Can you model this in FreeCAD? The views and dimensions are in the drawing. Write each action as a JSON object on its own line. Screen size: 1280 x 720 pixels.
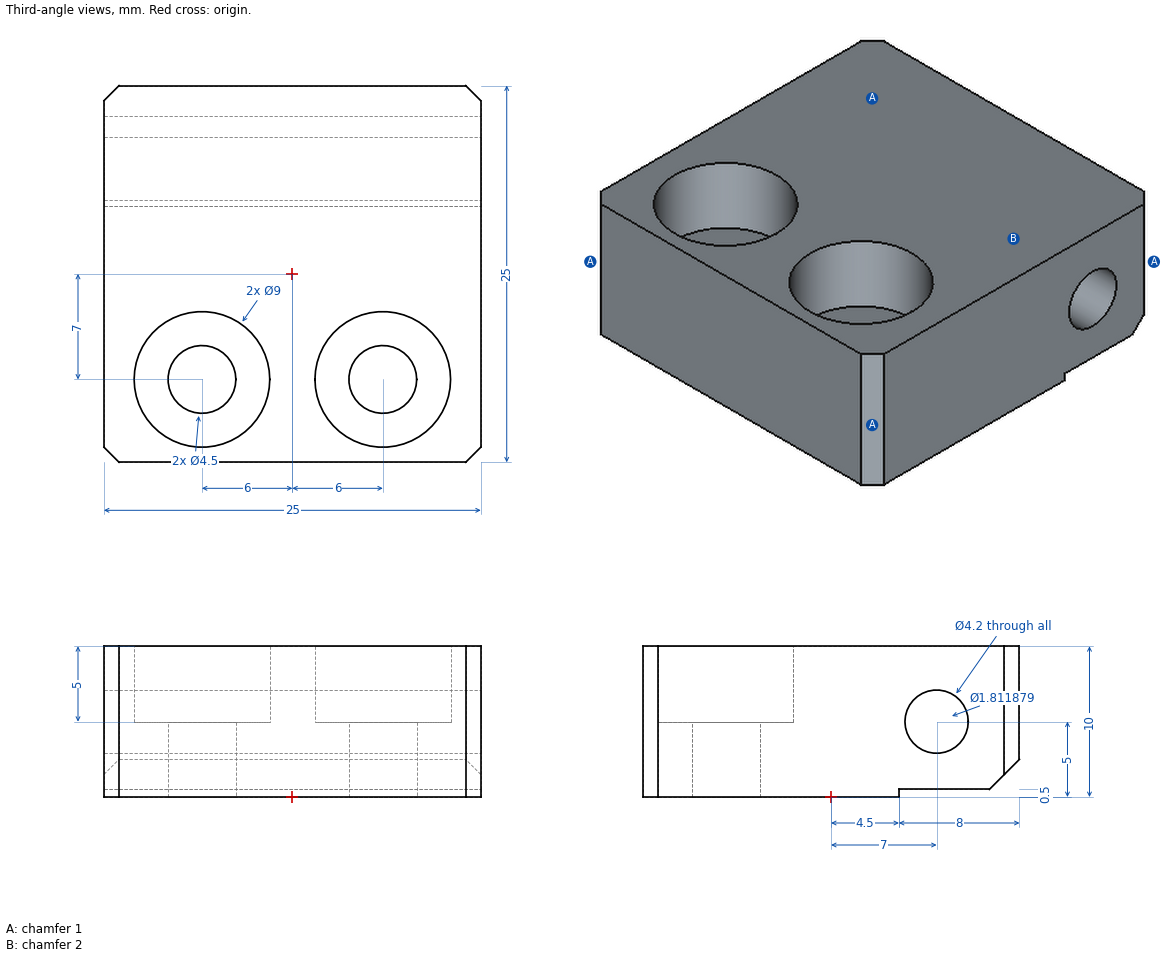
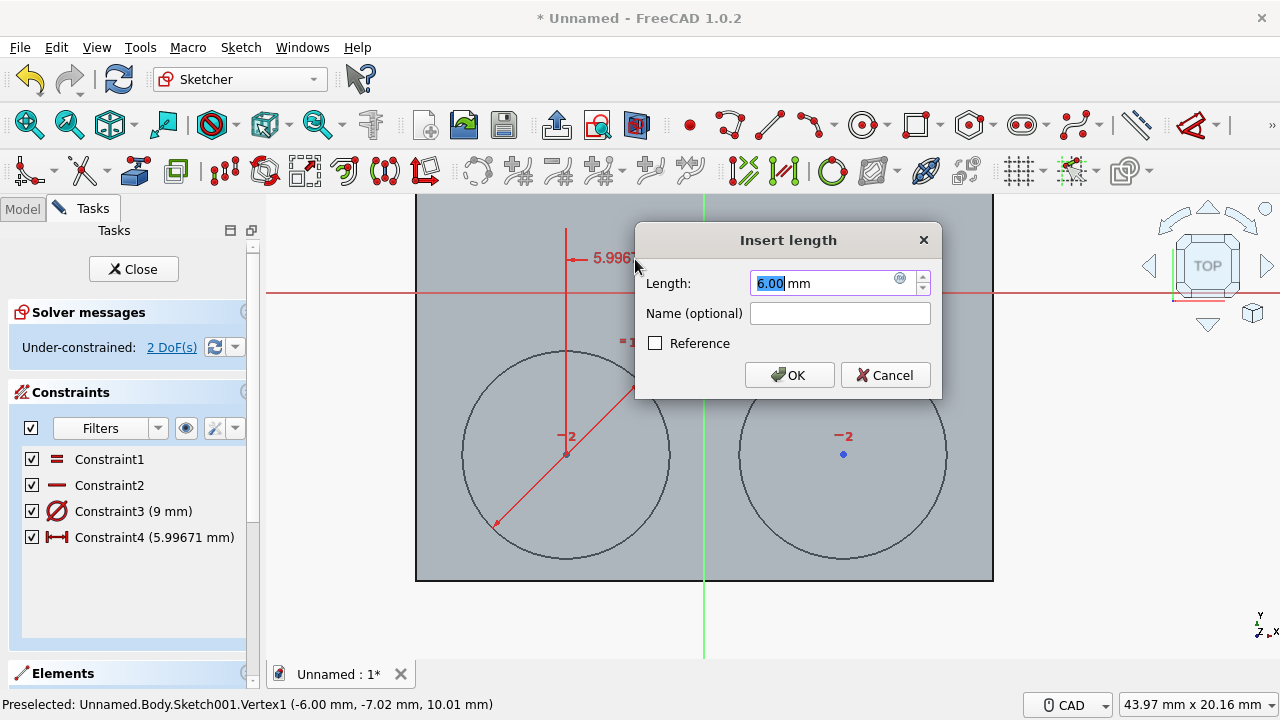
{"action": "type", "text": "6"}
{"action": "key", "text": "Return"}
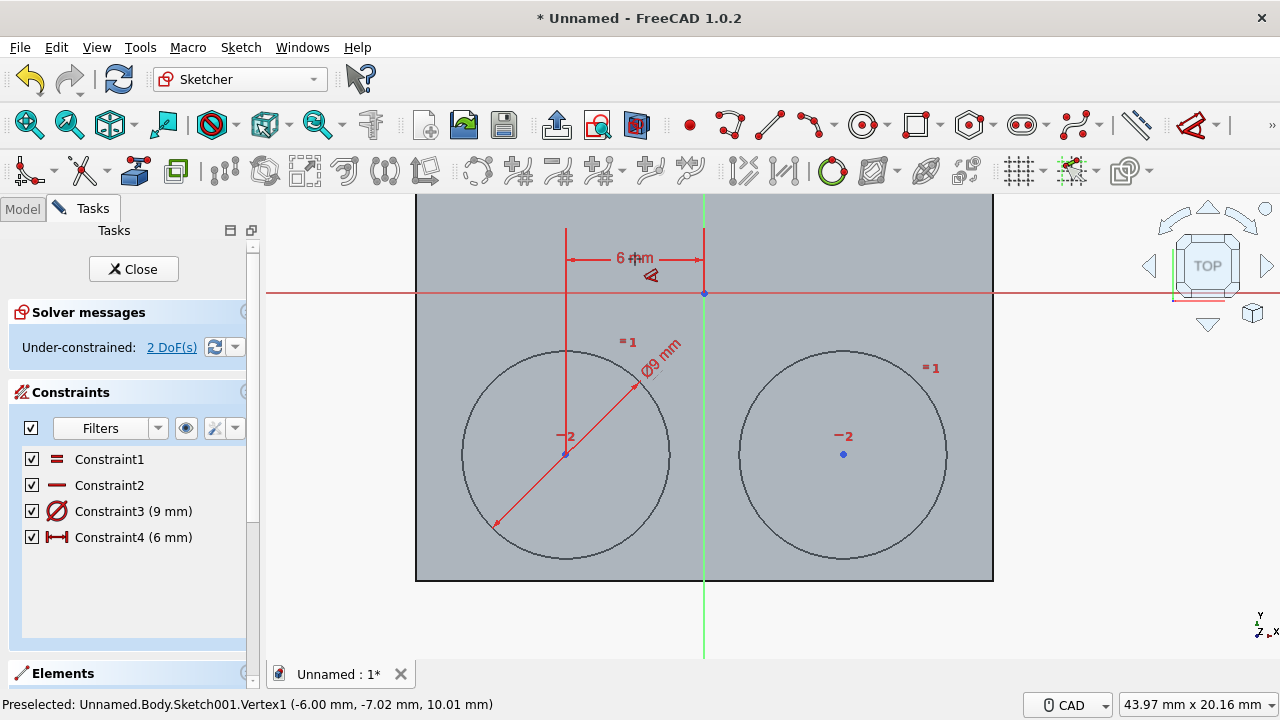
{"action": "left_click", "coordinate": [566, 455]}
{"action": "left_click", "coordinate": [532, 374]}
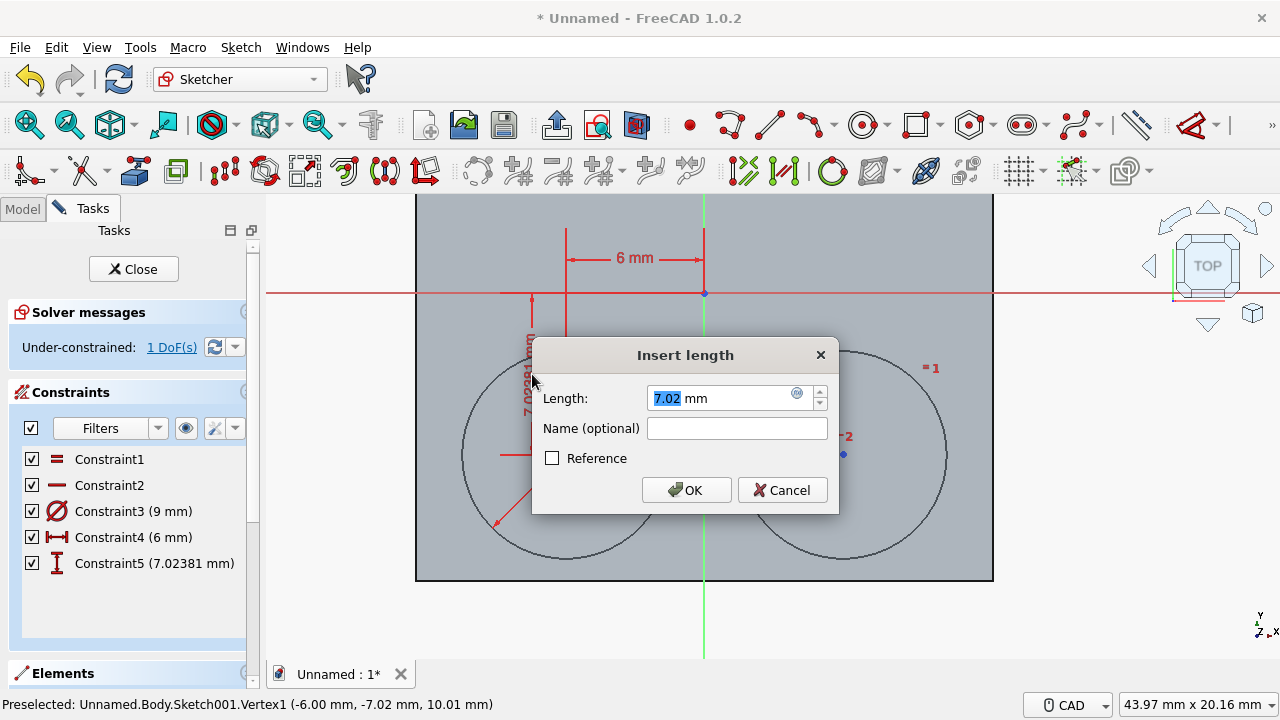
{"action": "type", "text": "7"}
{"action": "key", "text": "Return"}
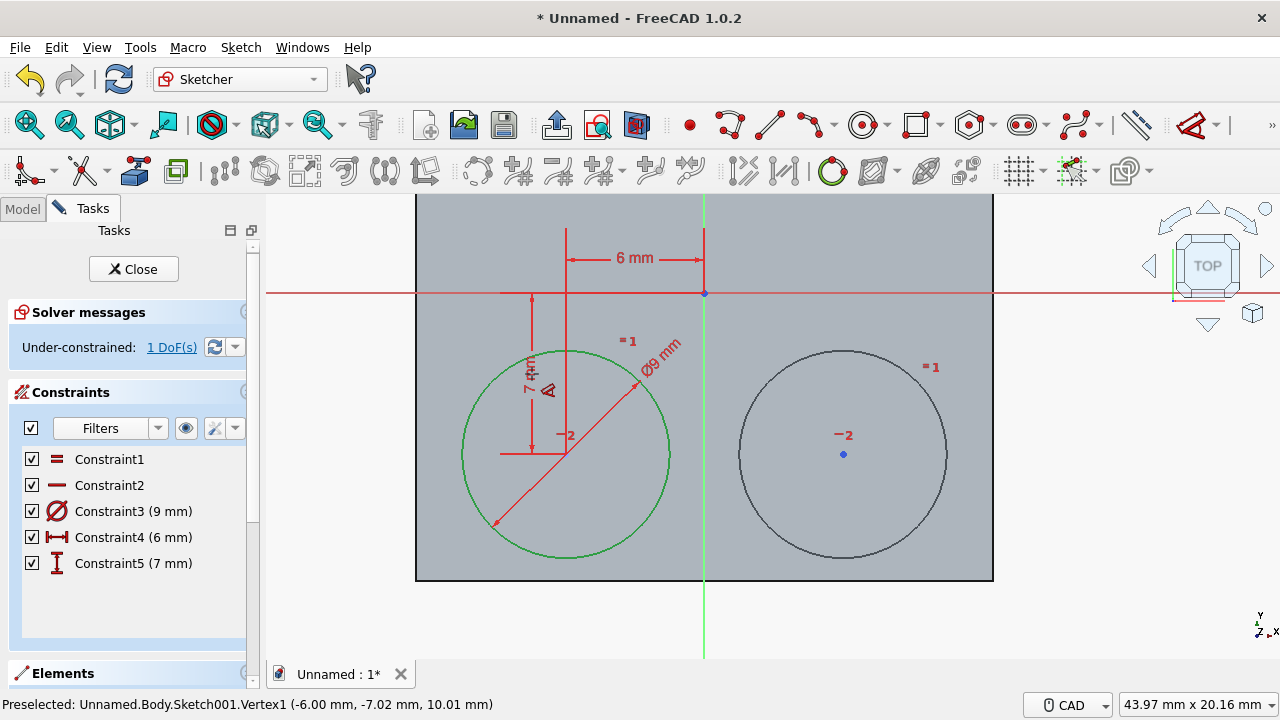
{"action": "left_click", "coordinate": [843, 454]}
{"action": "left_click", "coordinate": [774, 259]}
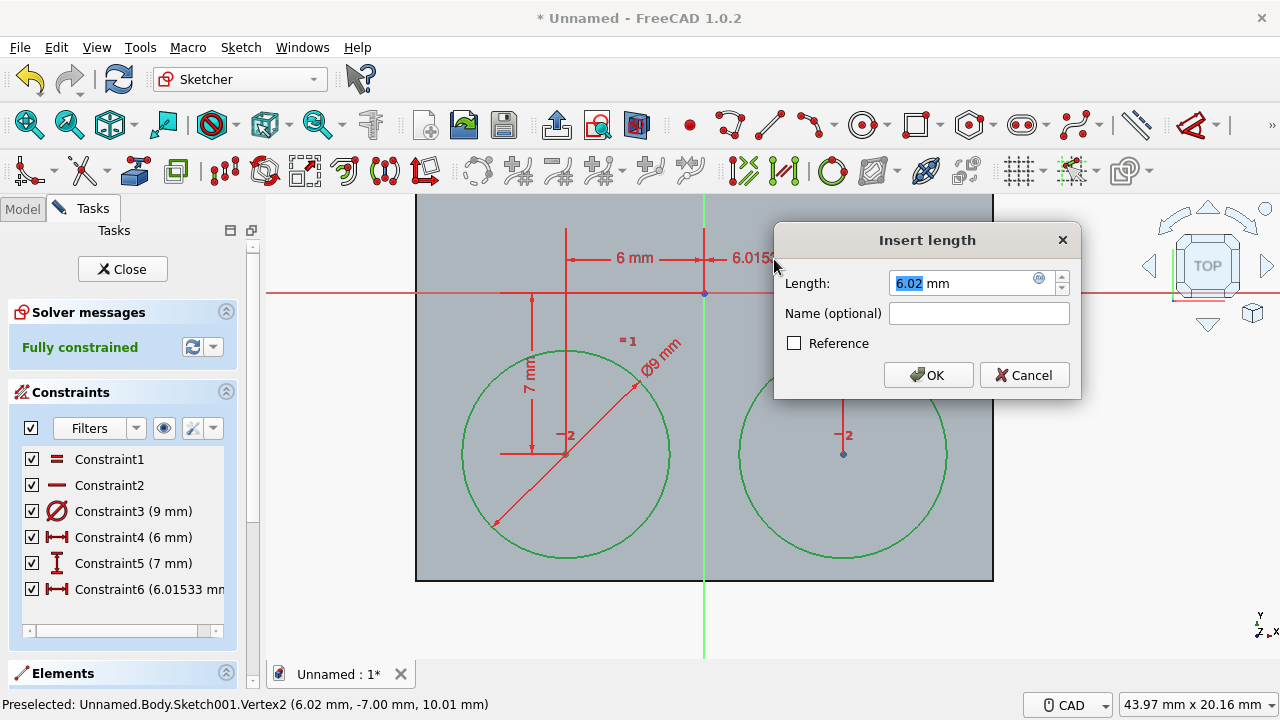
{"action": "type", "text": "6"}
{"action": "key", "text": "Return"}
{"action": "key", "text": "Escape"}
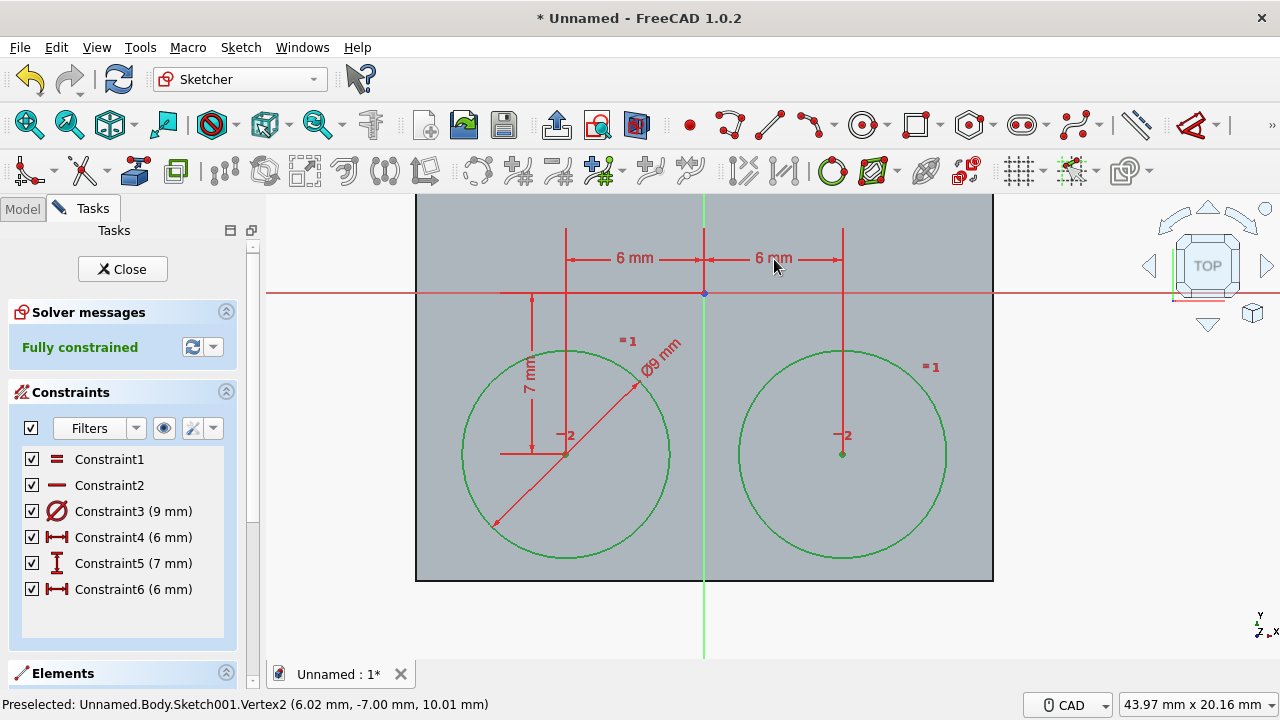
{"action": "left_click", "coordinate": [123, 269]}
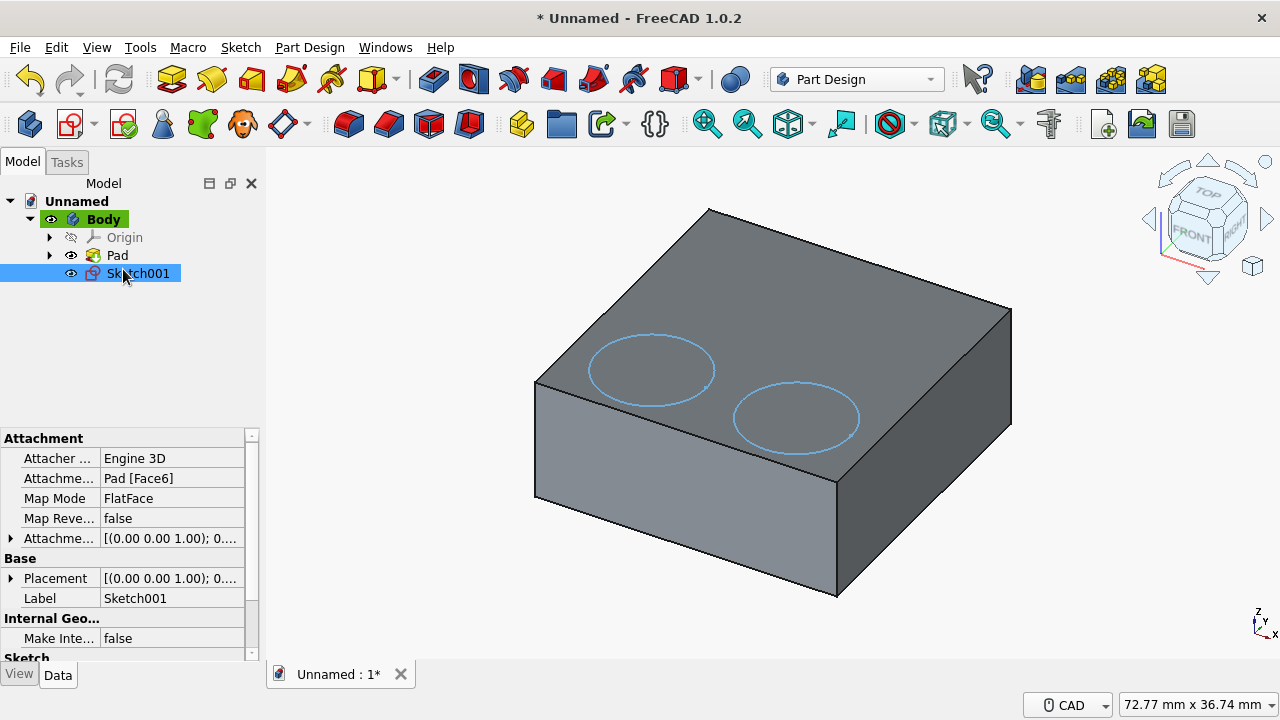
{"action": "left_click", "coordinate": [434, 80]}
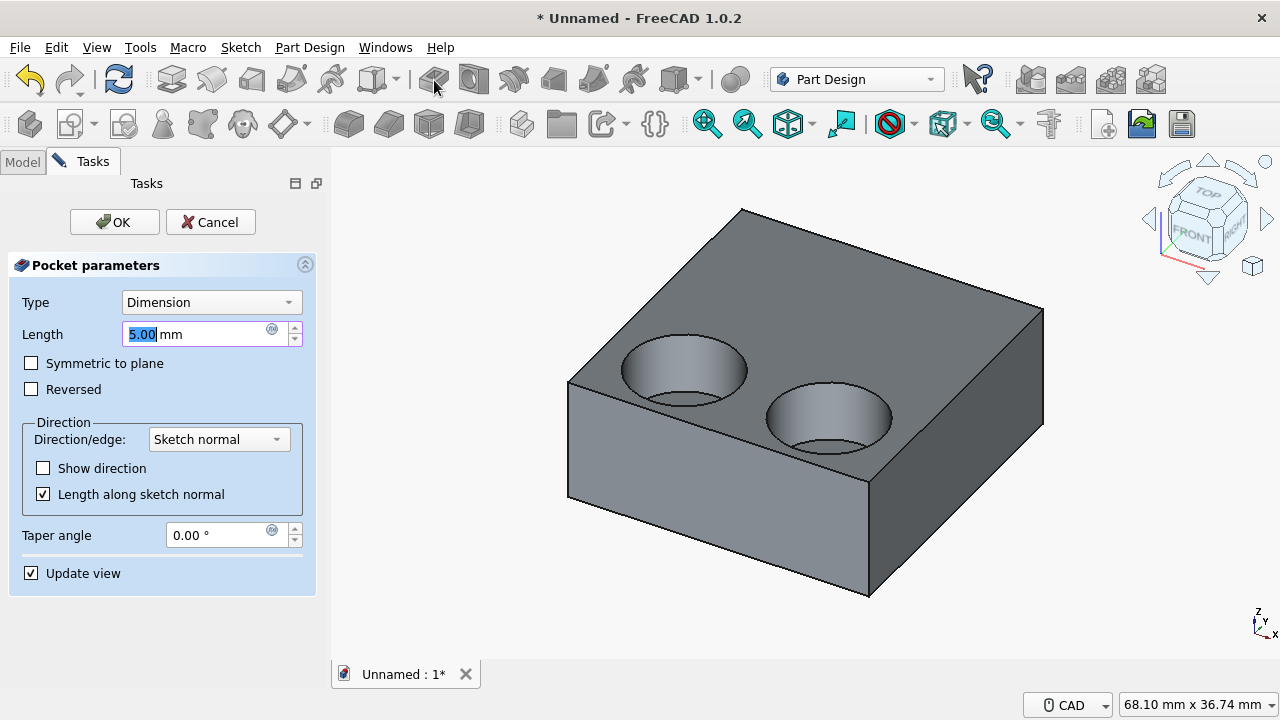
{"action": "type", "text": "5"}
{"action": "key", "text": "Tab"}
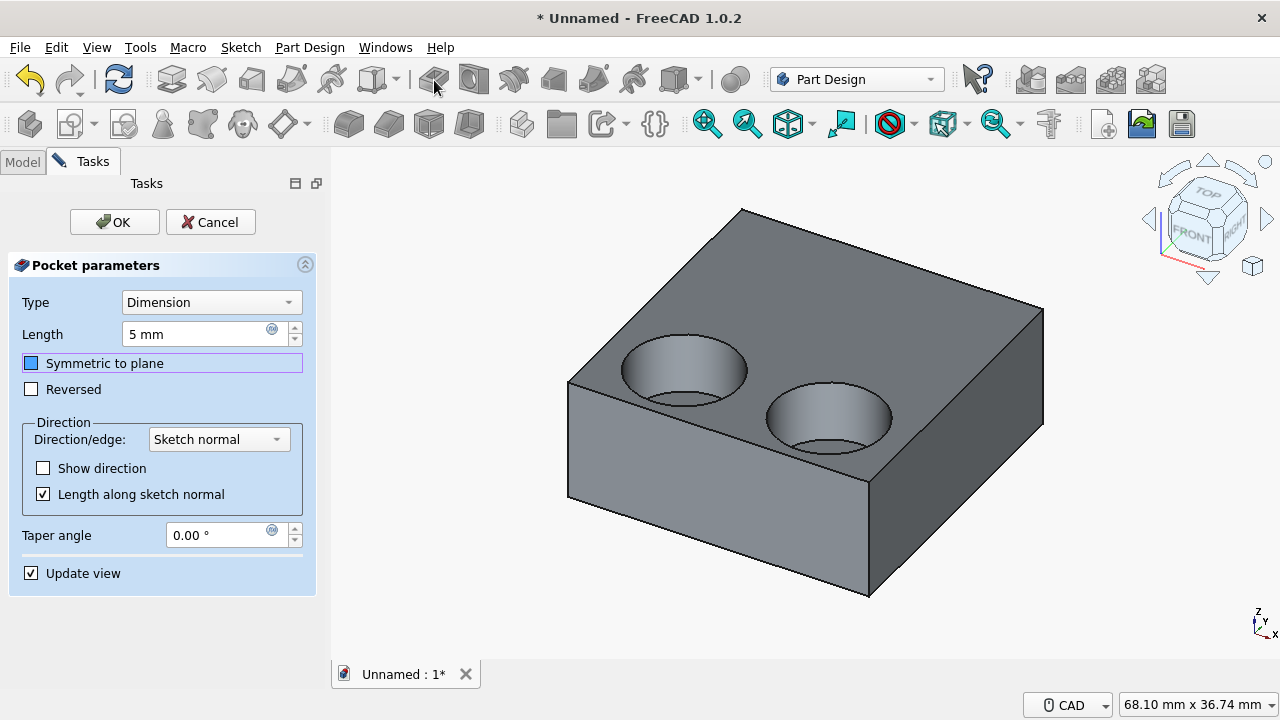
{"action": "left_click", "coordinate": [115, 222]}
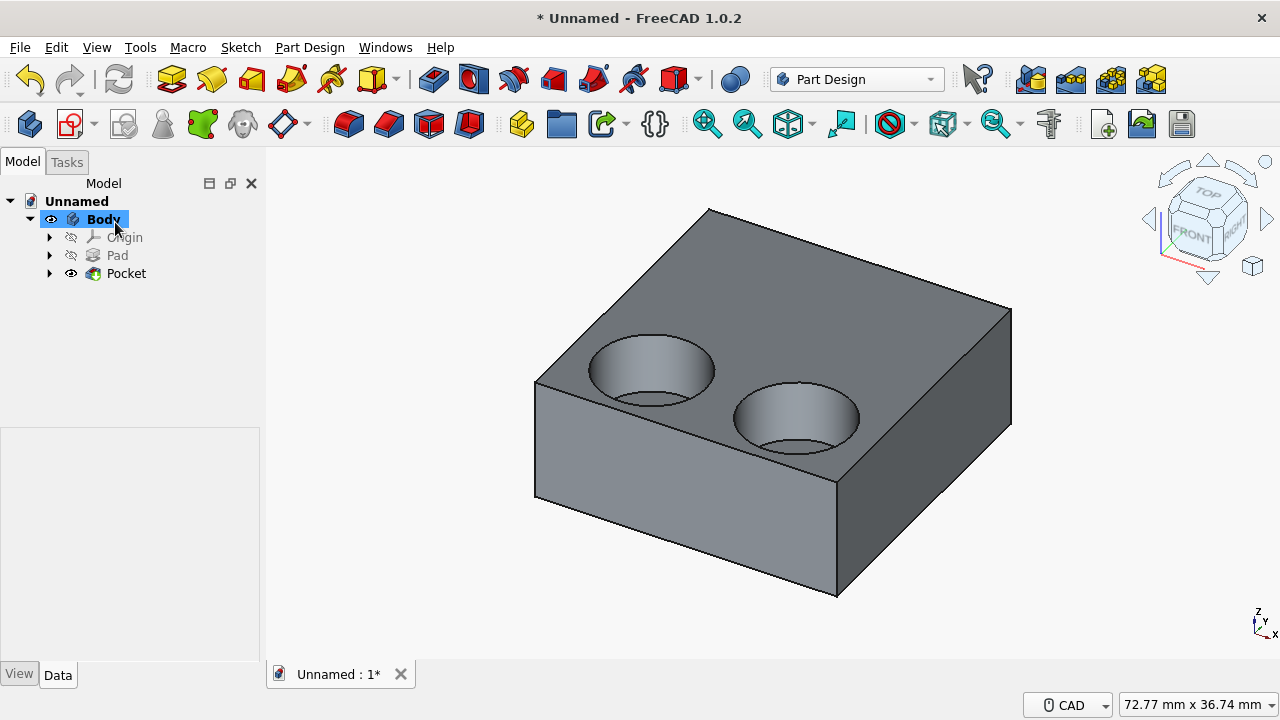
{"action": "left_click", "coordinate": [798, 320]}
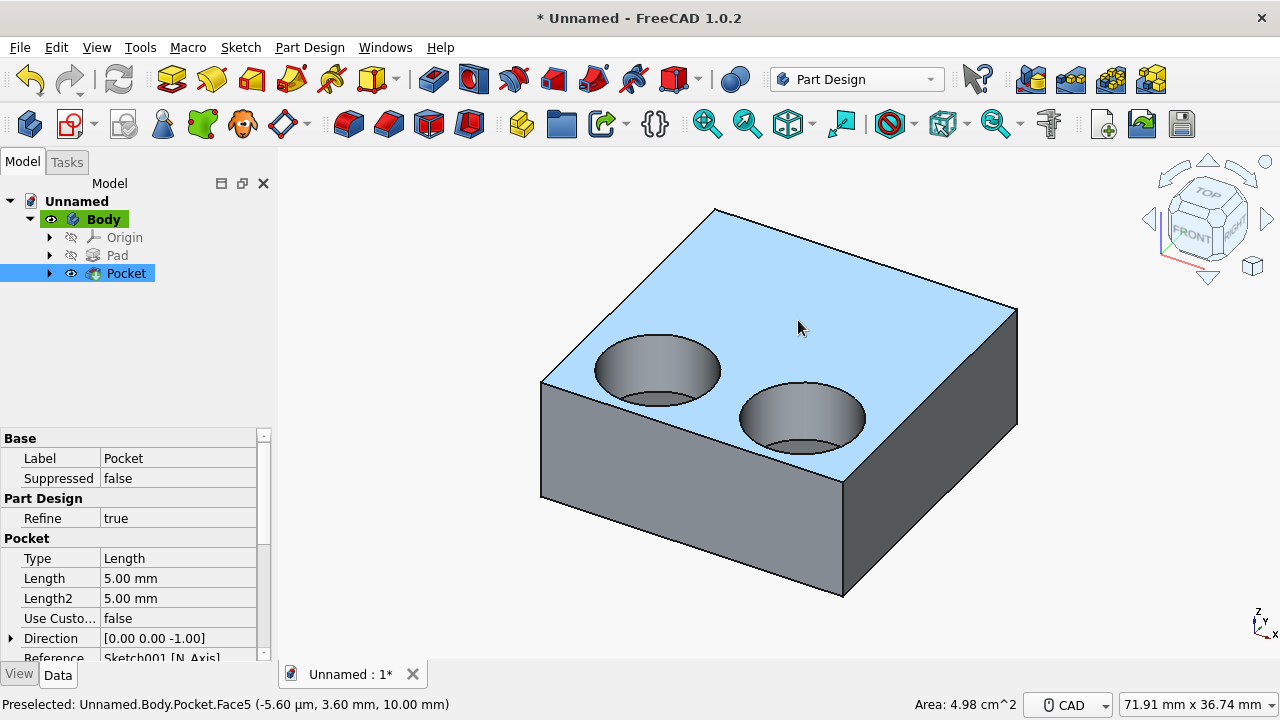
{"action": "left_click", "coordinate": [70, 124]}